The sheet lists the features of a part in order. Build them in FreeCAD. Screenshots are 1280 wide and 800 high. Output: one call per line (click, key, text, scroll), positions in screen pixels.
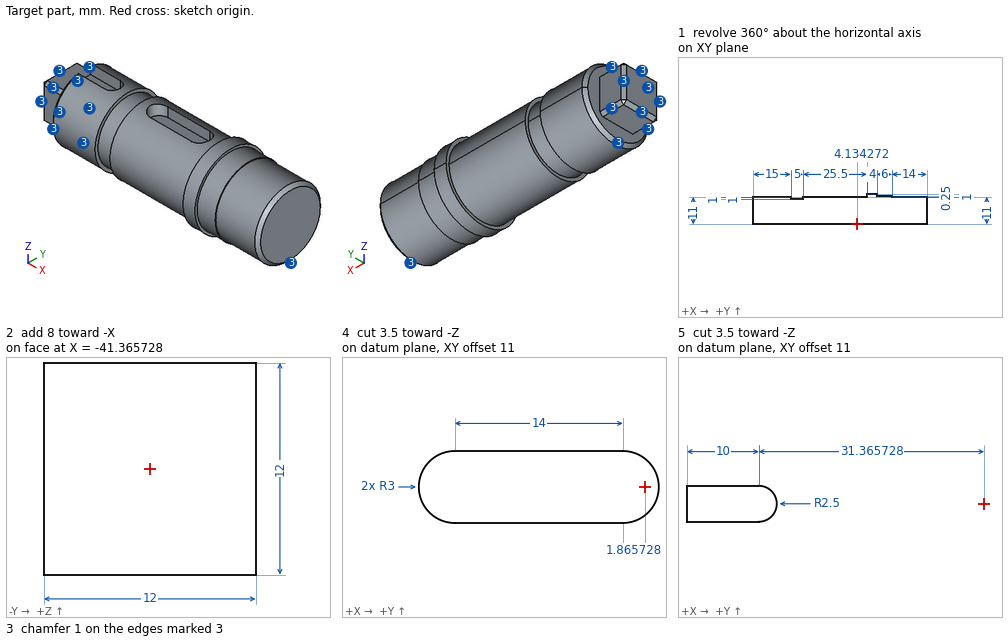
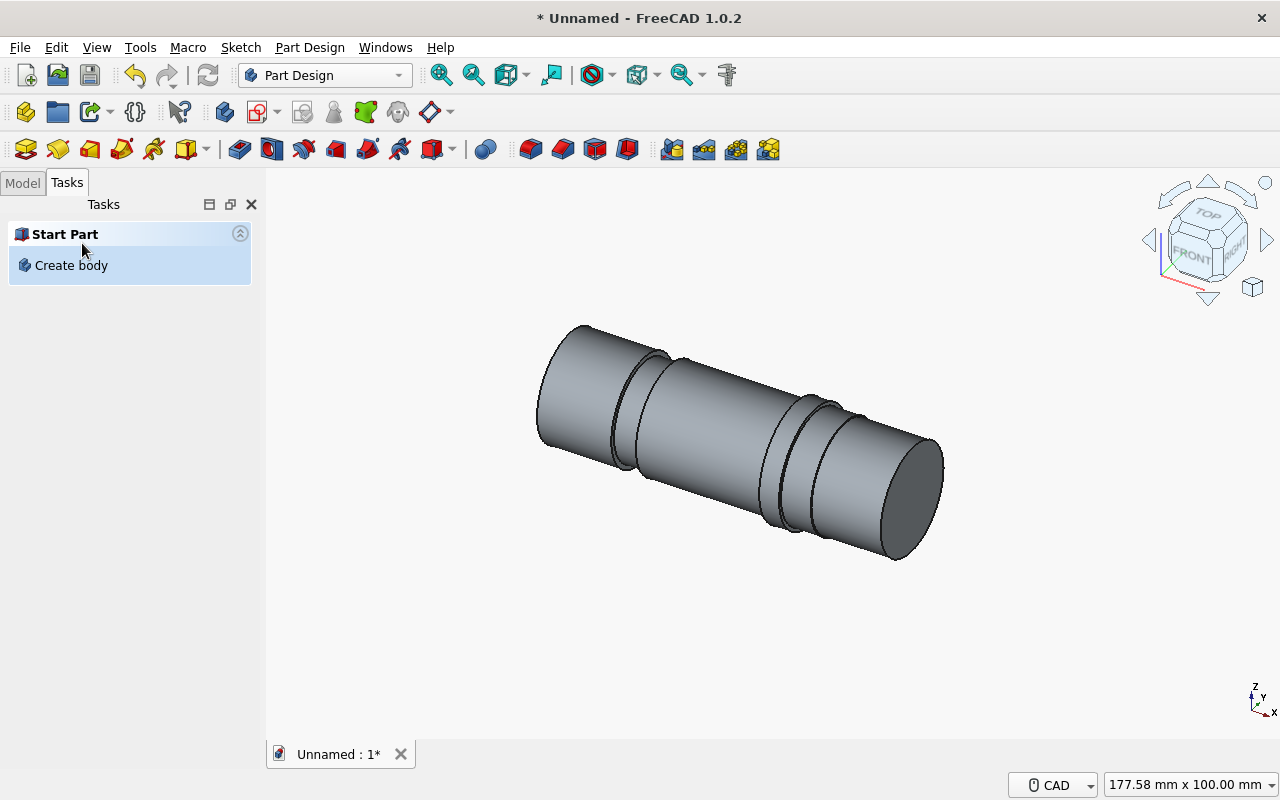
key(6)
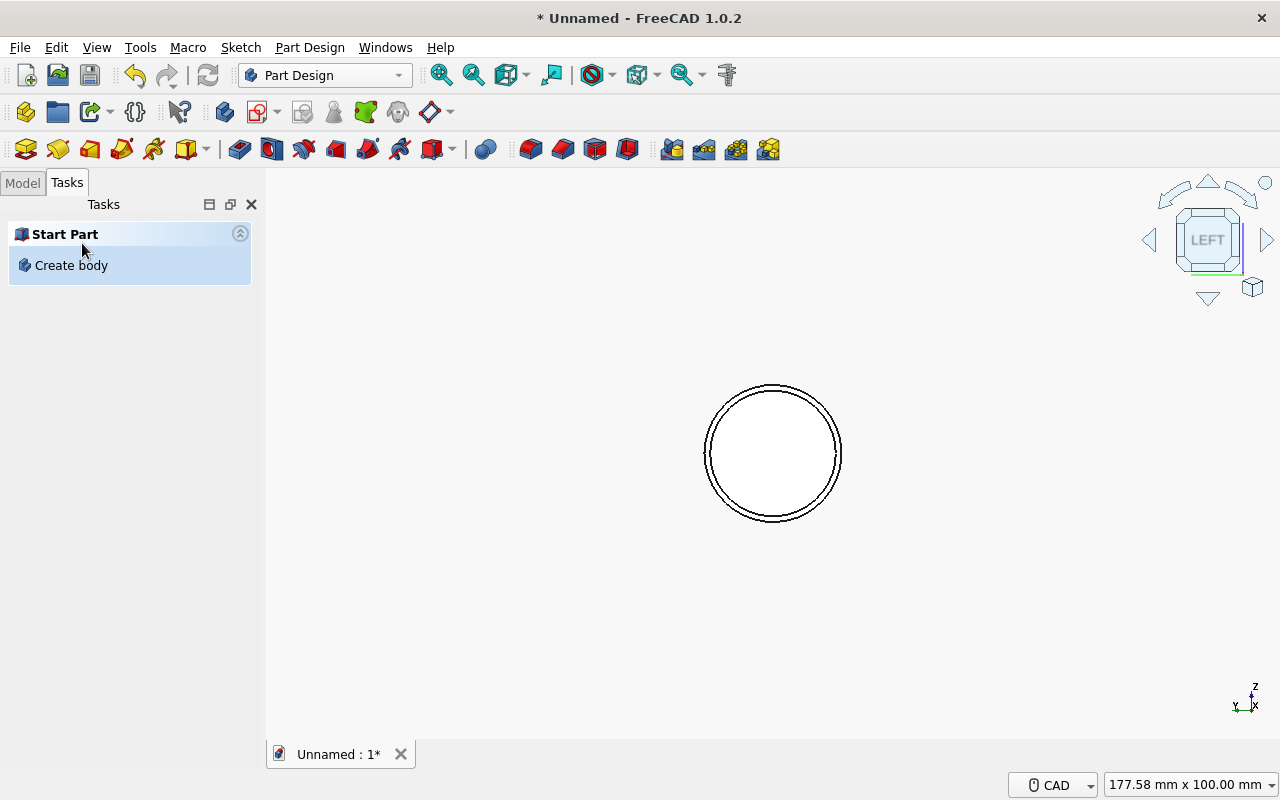
click(442, 76)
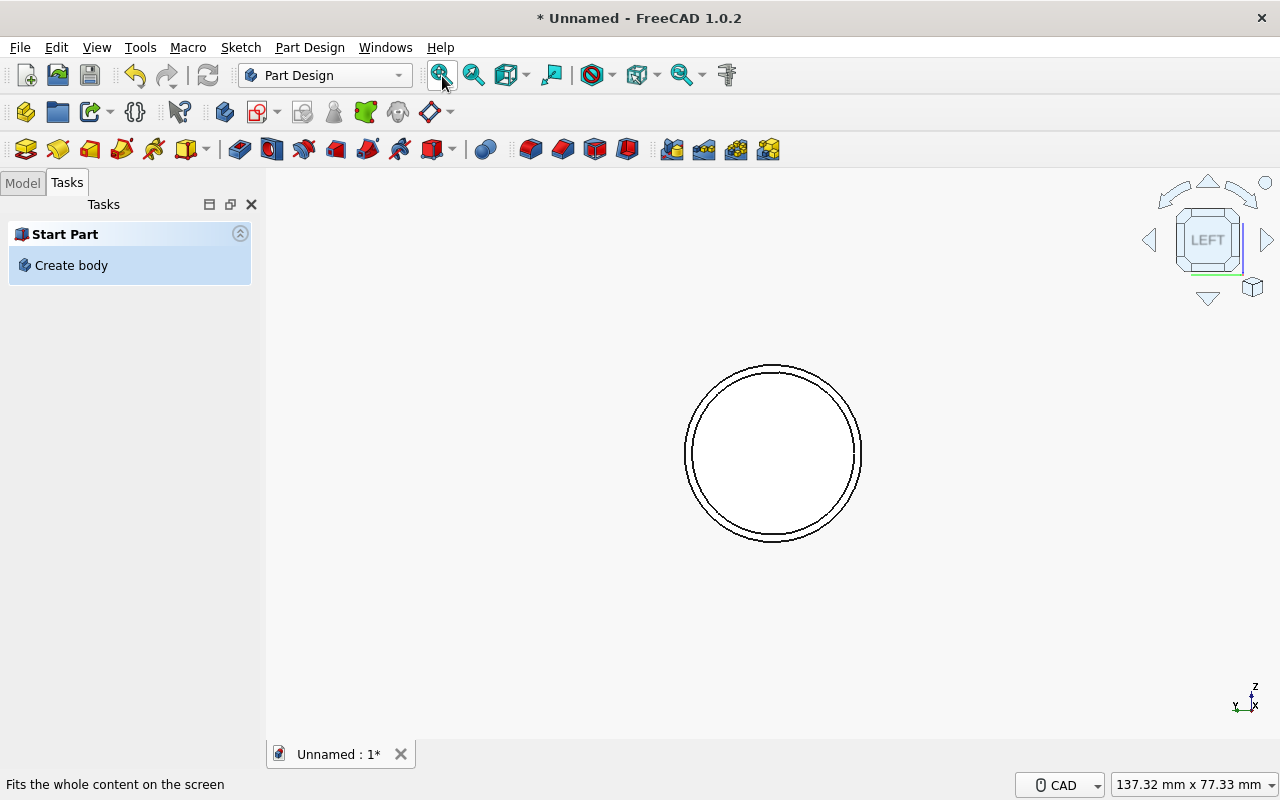
click(773, 452)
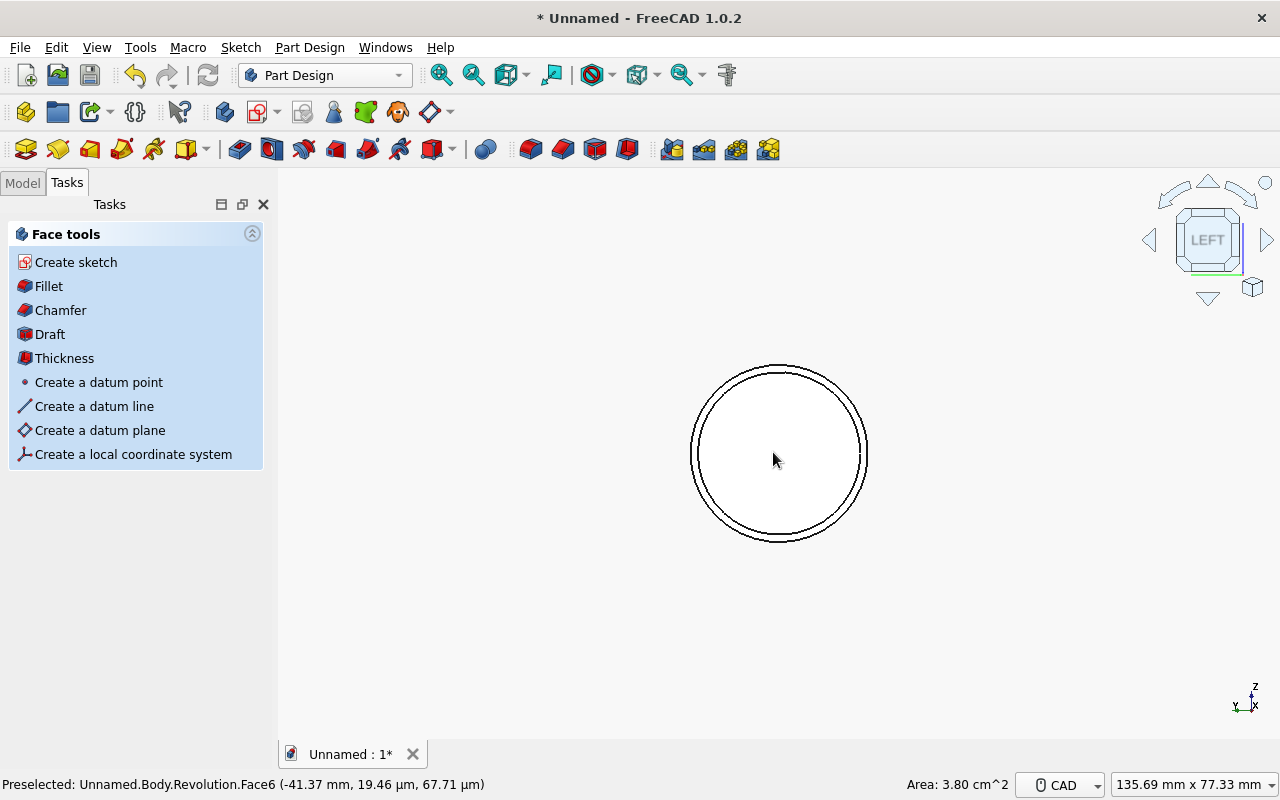
click(258, 112)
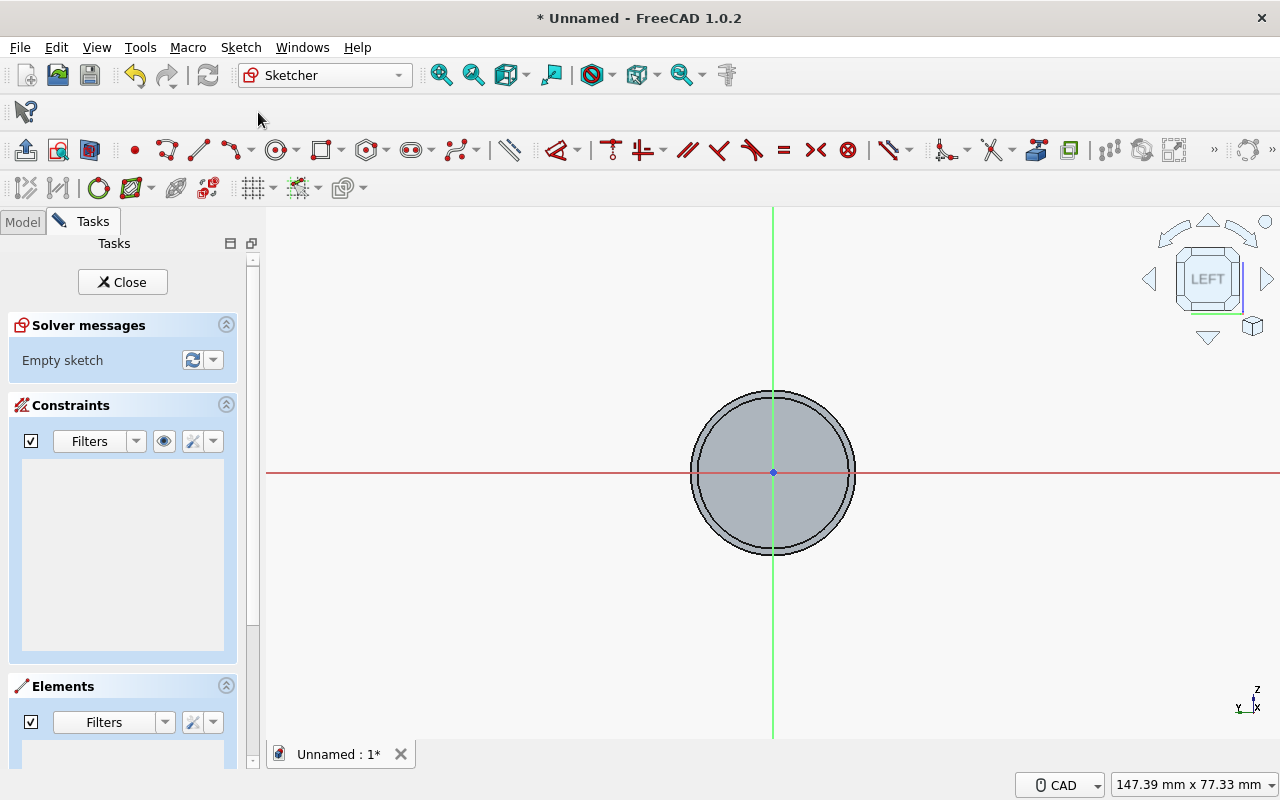
scroll(796, 473, up, 7)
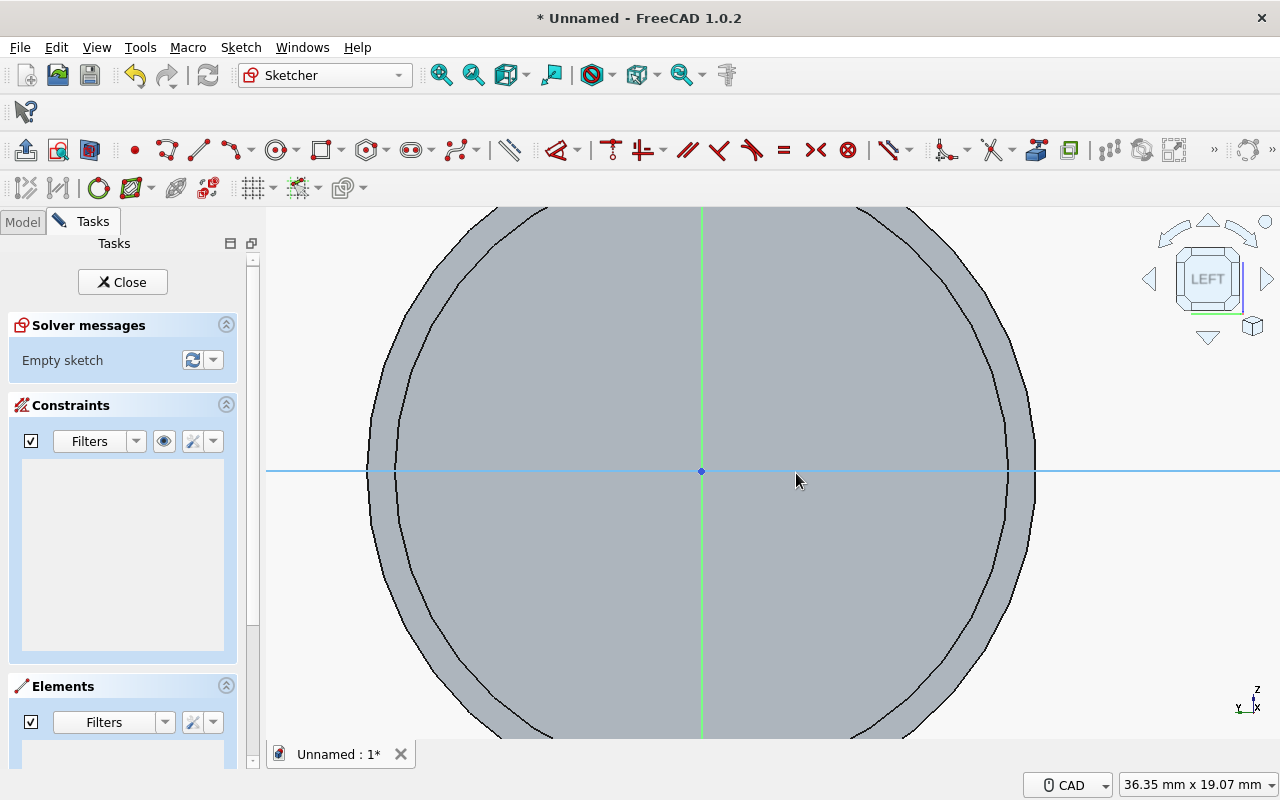
click(344, 150)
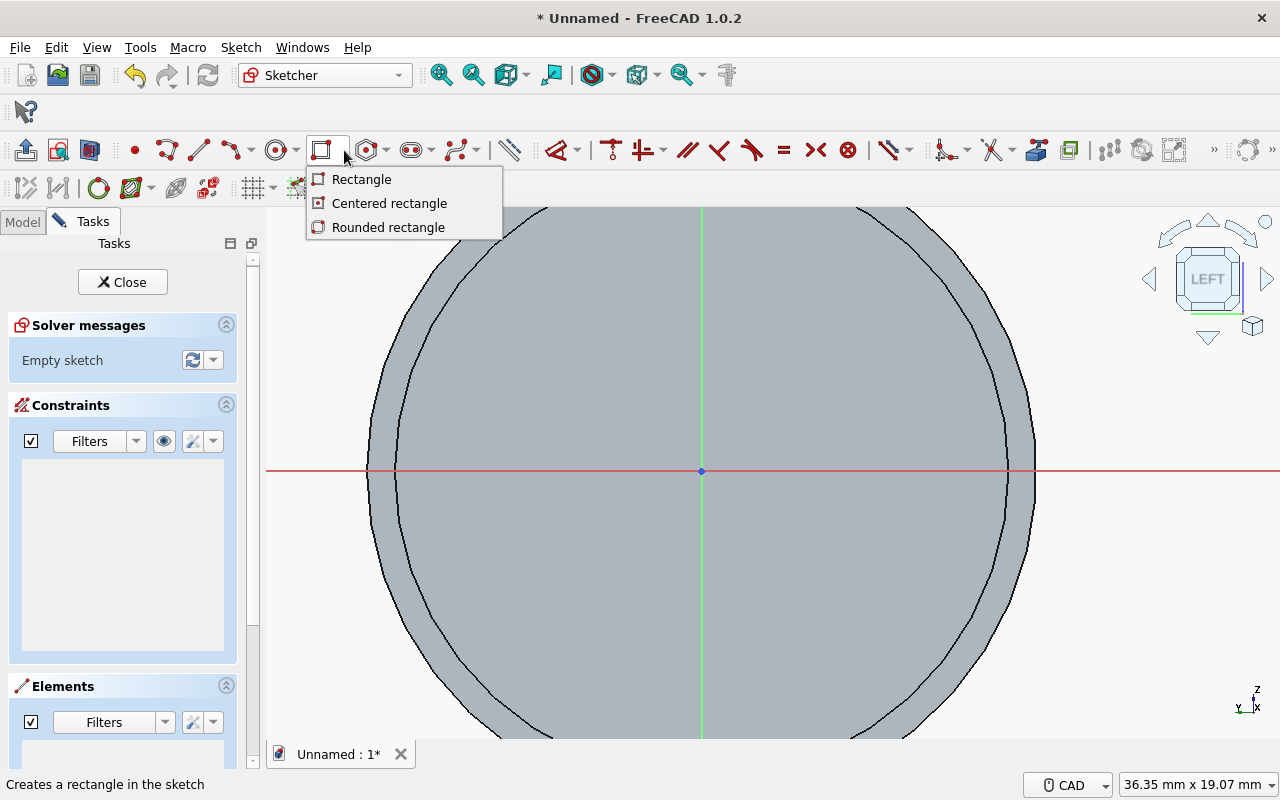
click(404, 203)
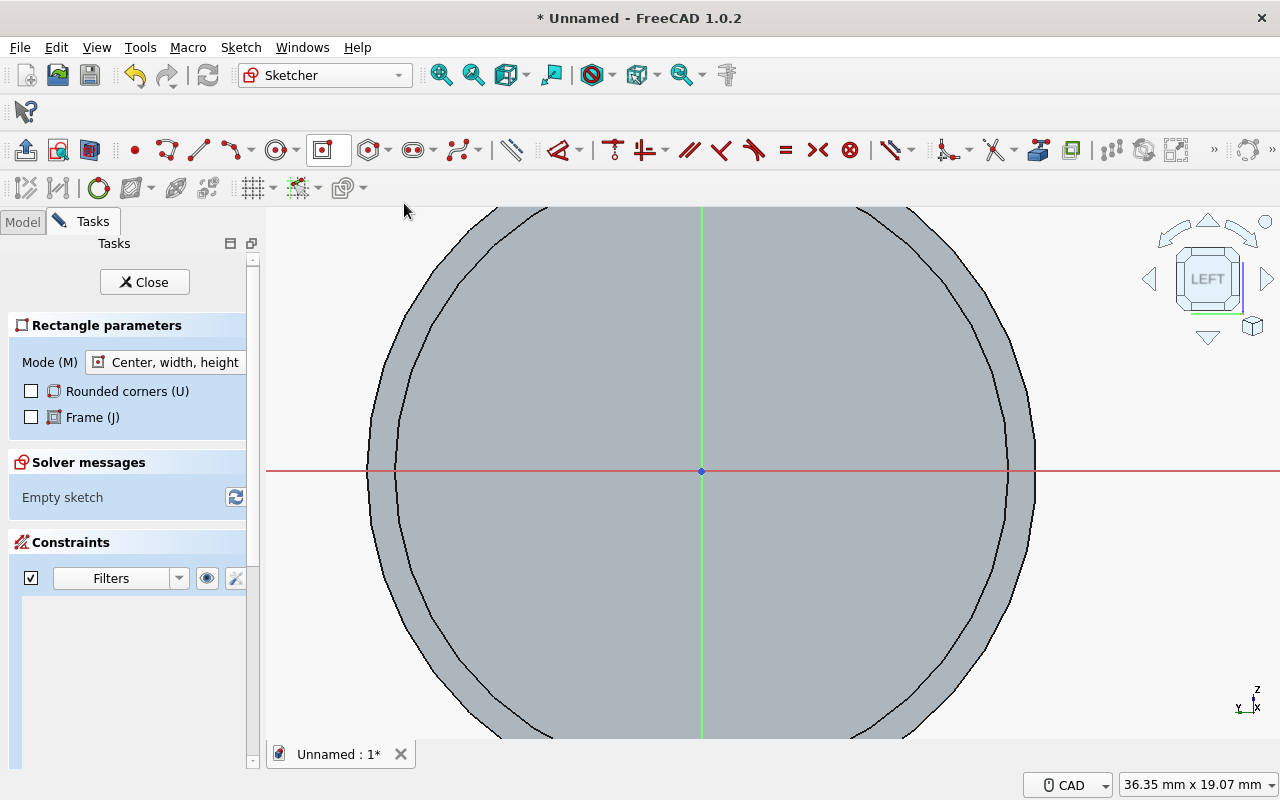
click(702, 471)
move(869, 304)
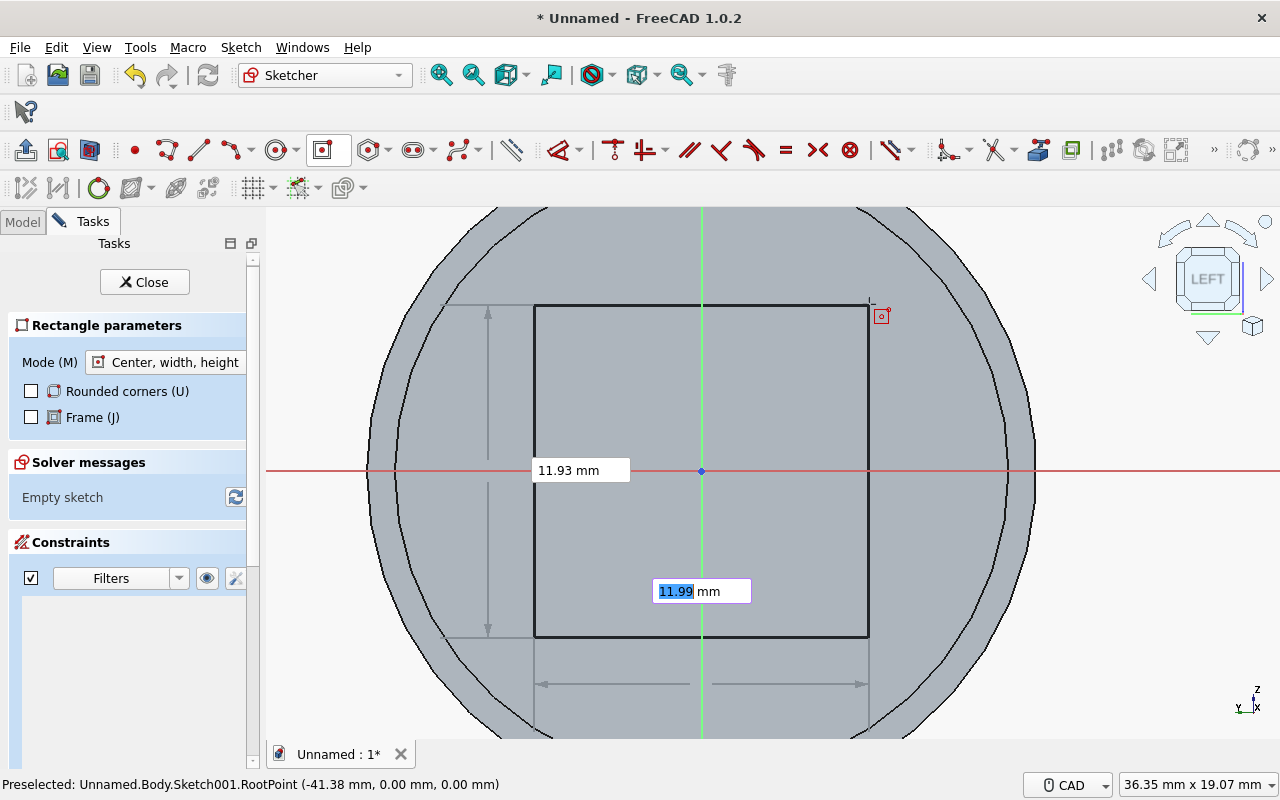
text(12)
key(Tab)
text(12)
key(Return)
key(Escape)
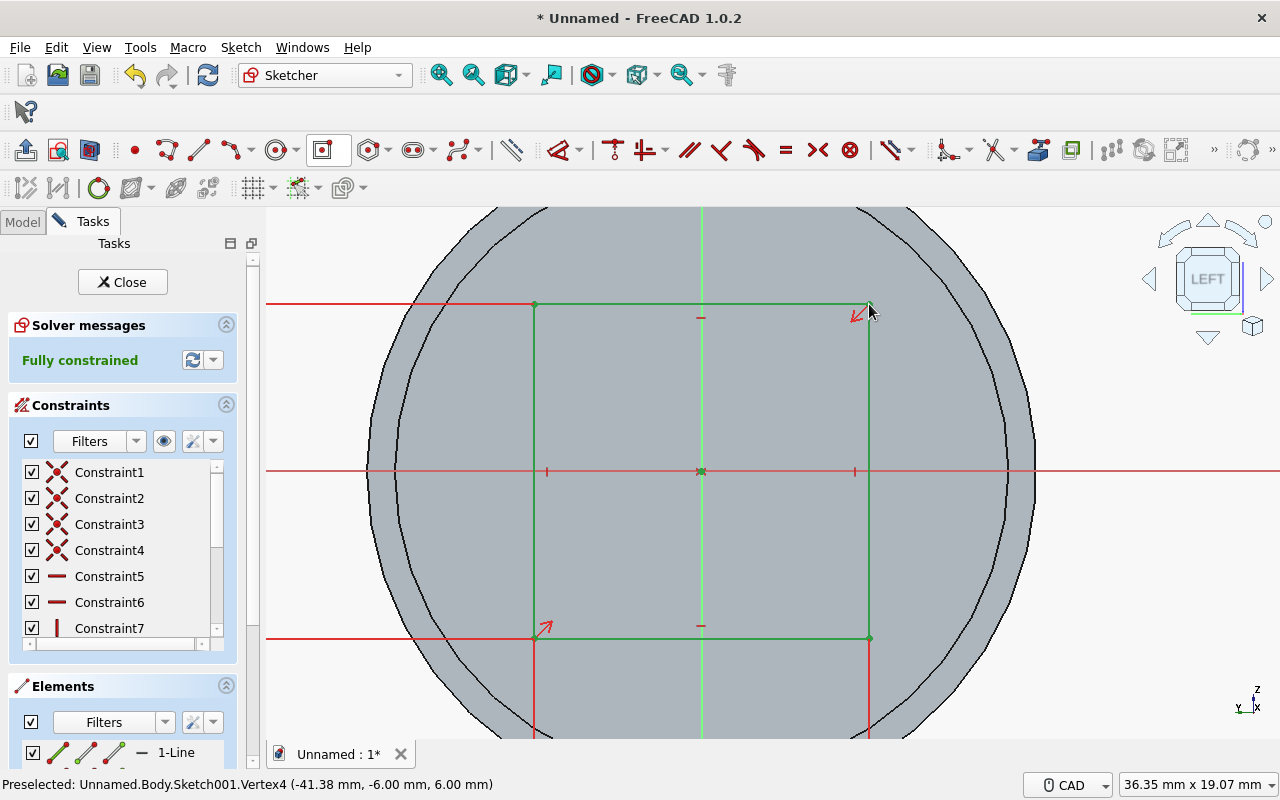
click(123, 282)